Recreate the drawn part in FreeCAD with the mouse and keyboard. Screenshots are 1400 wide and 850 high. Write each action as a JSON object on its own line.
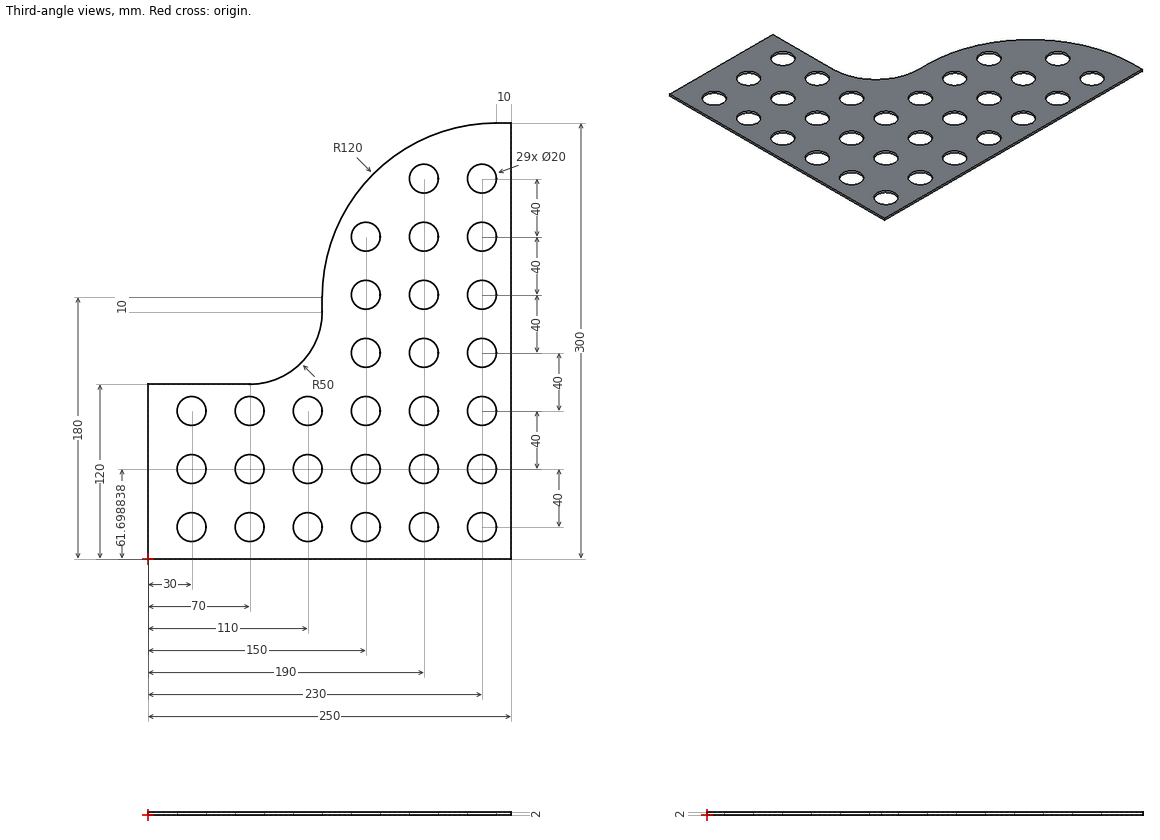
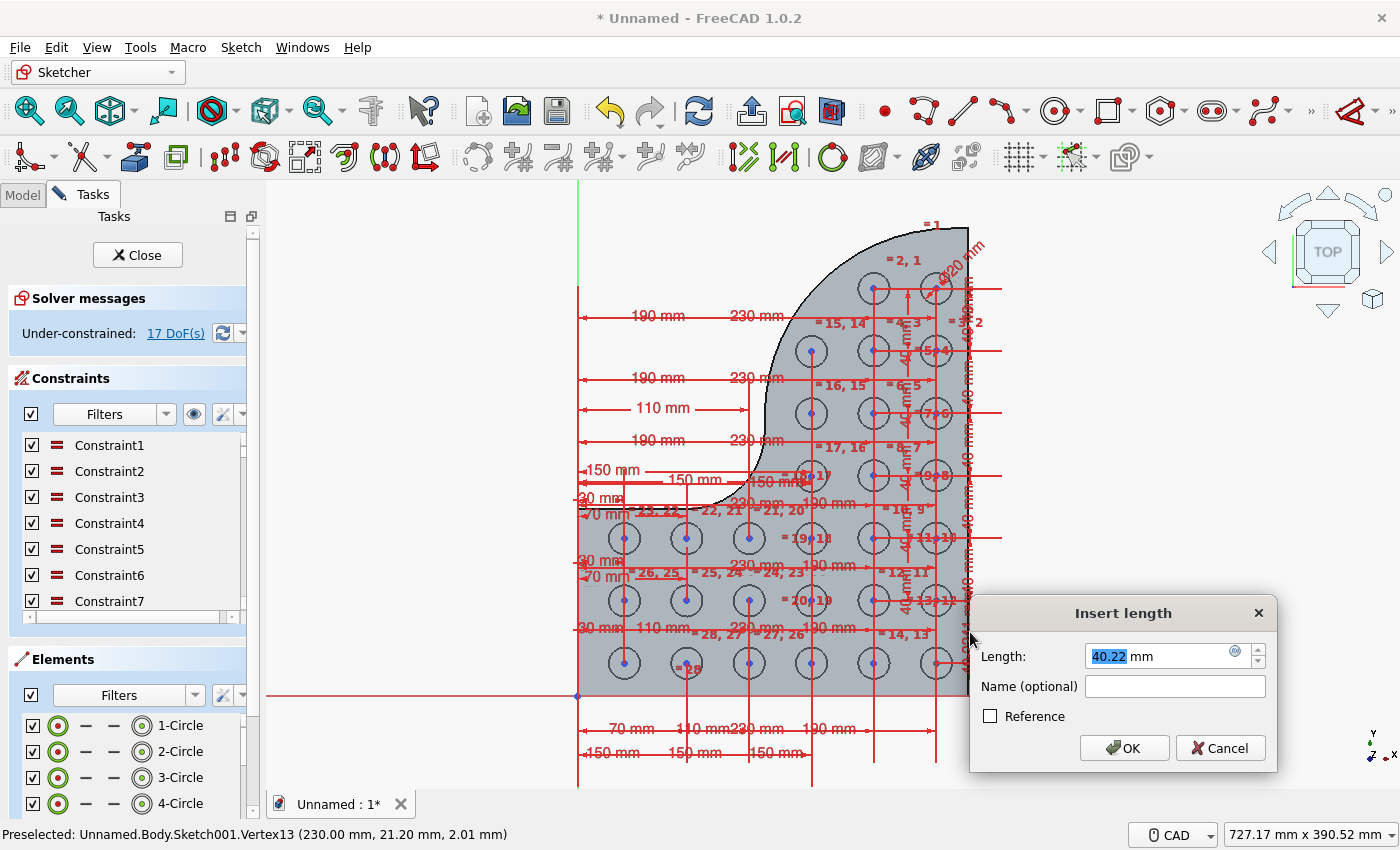
{"action": "type", "text": "40"}
{"action": "key", "text": "Return"}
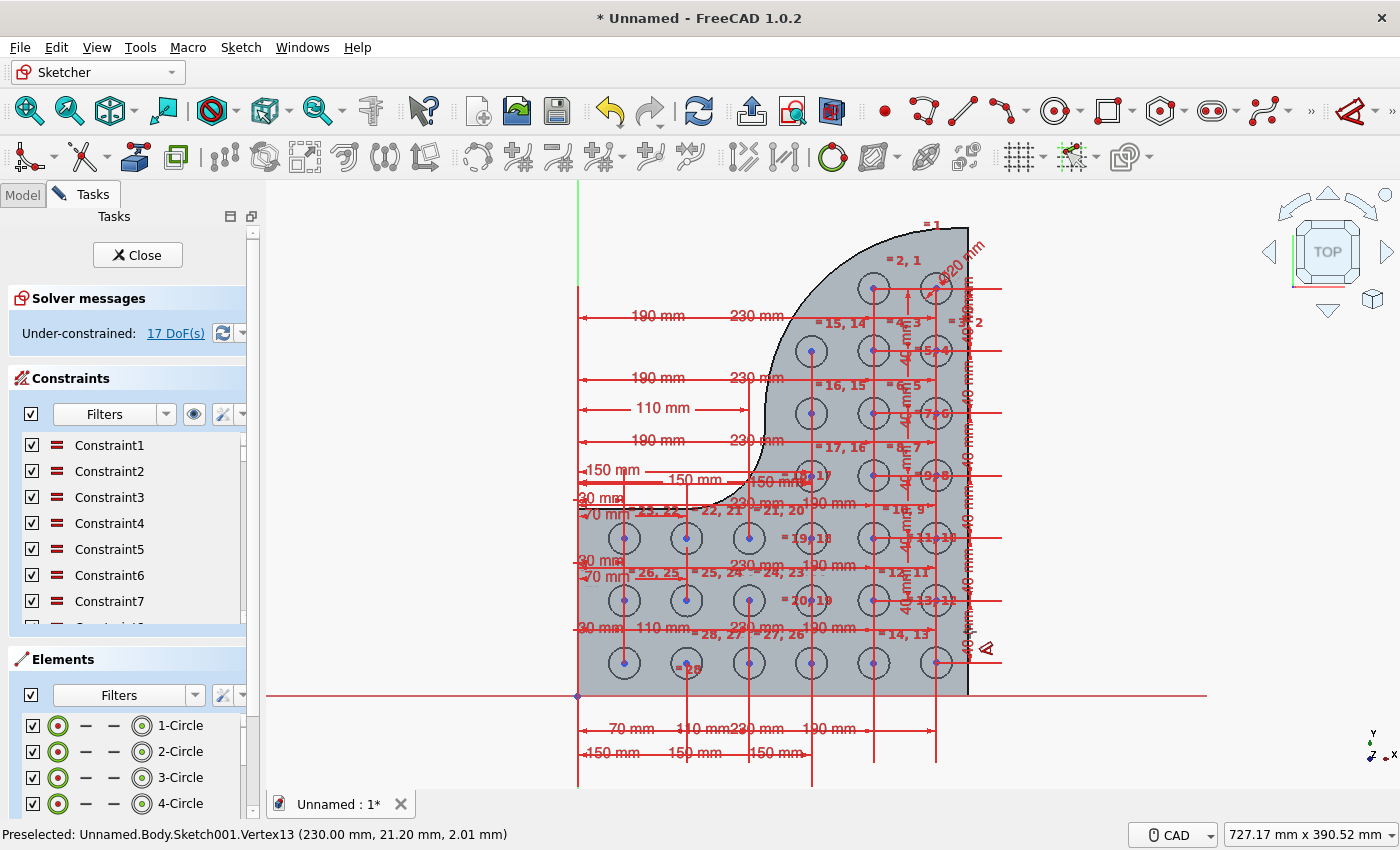
{"action": "left_click", "coordinate": [874, 601]}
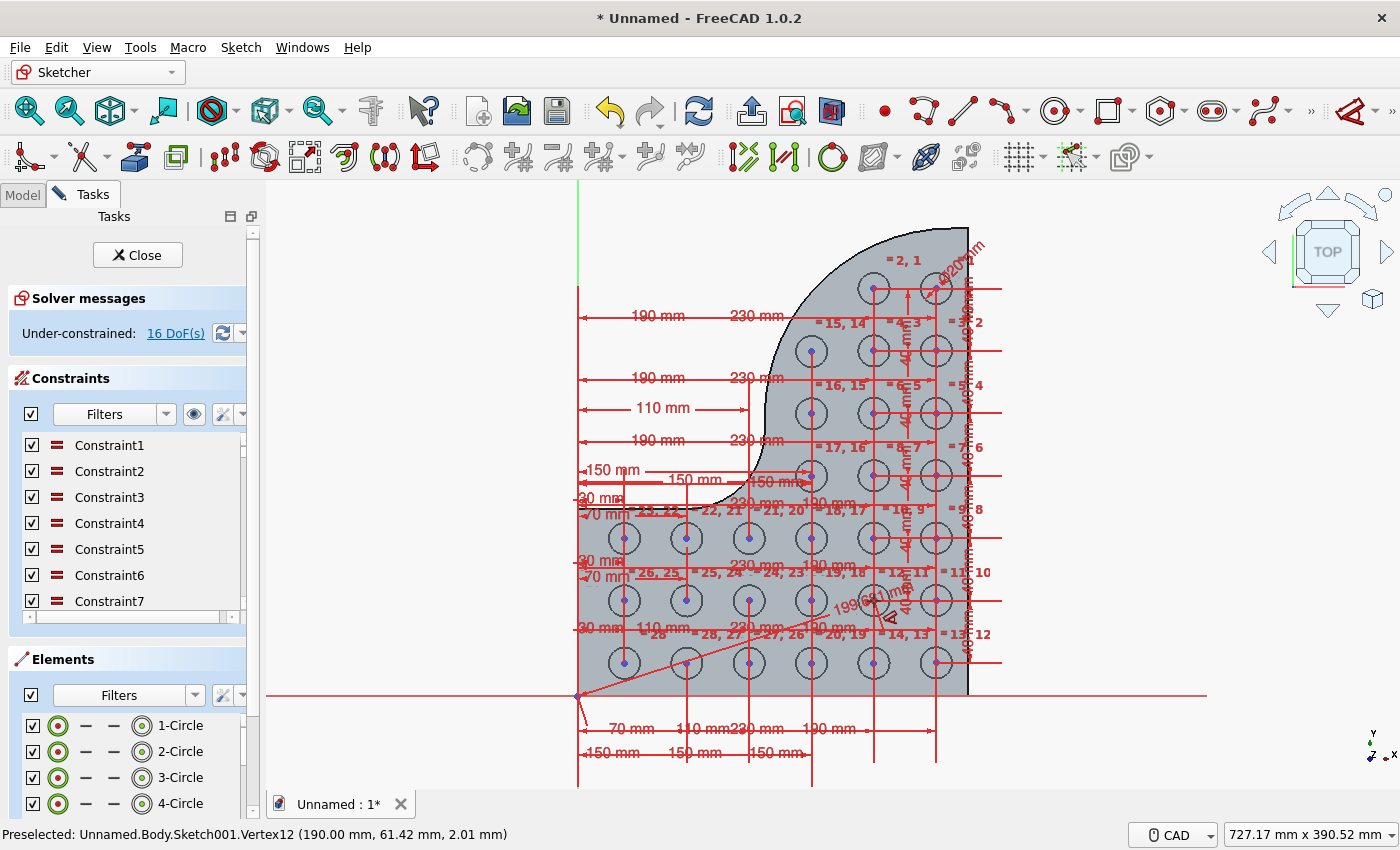
{"action": "left_click", "coordinate": [874, 663]}
{"action": "left_click", "coordinate": [908, 654]}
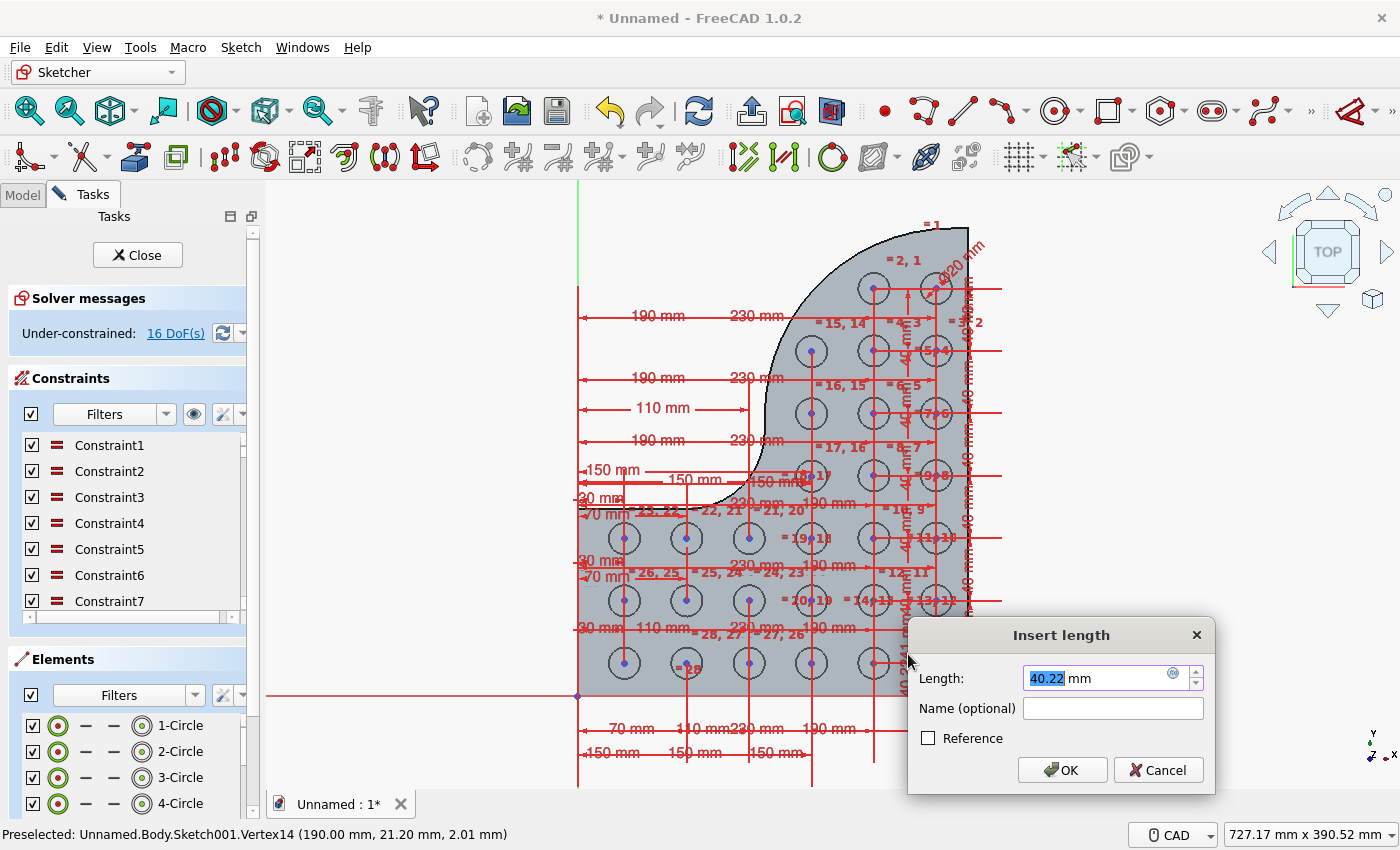
{"action": "type", "text": "40"}
{"action": "key", "text": "Return"}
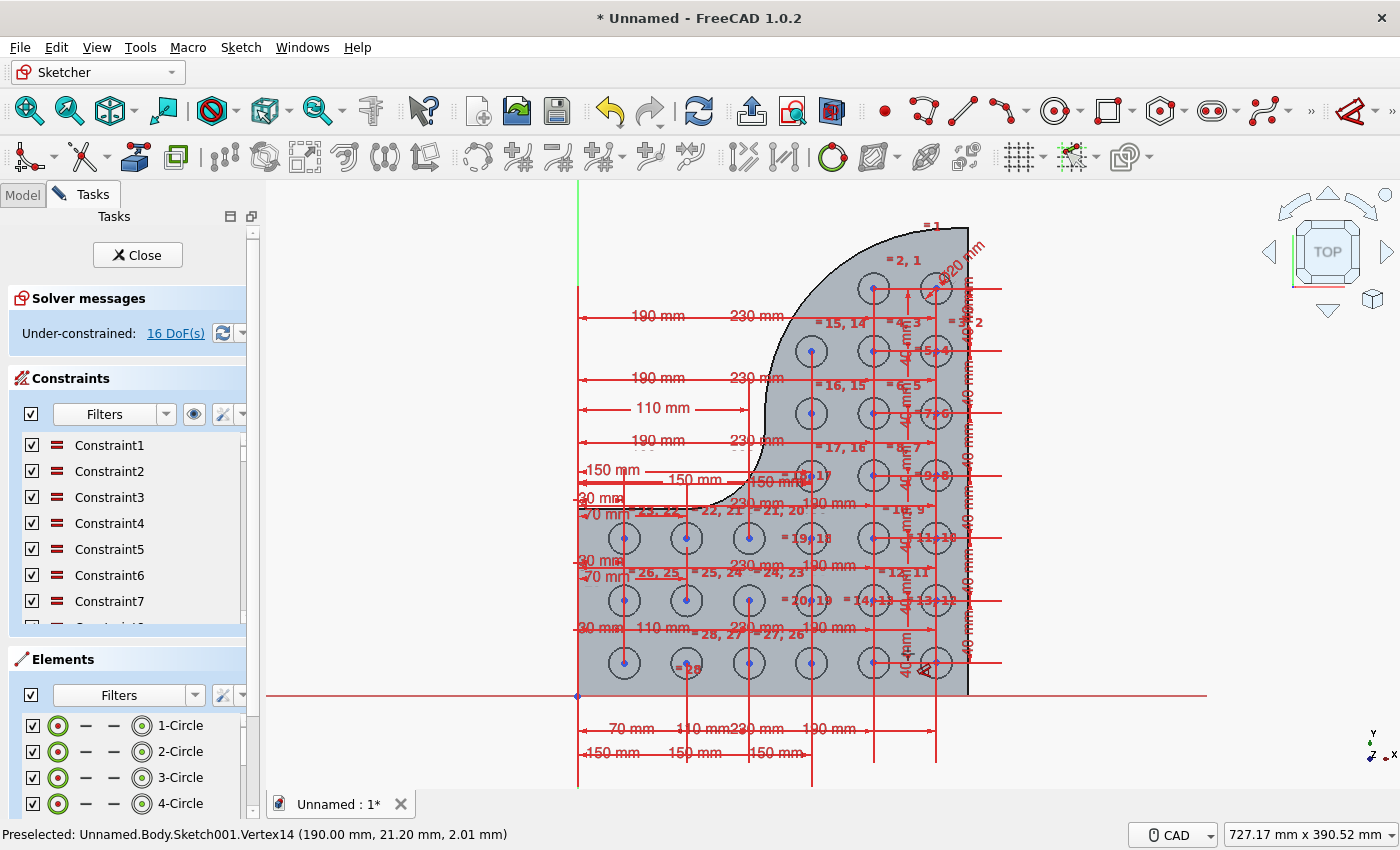
{"action": "left_click", "coordinate": [874, 289]}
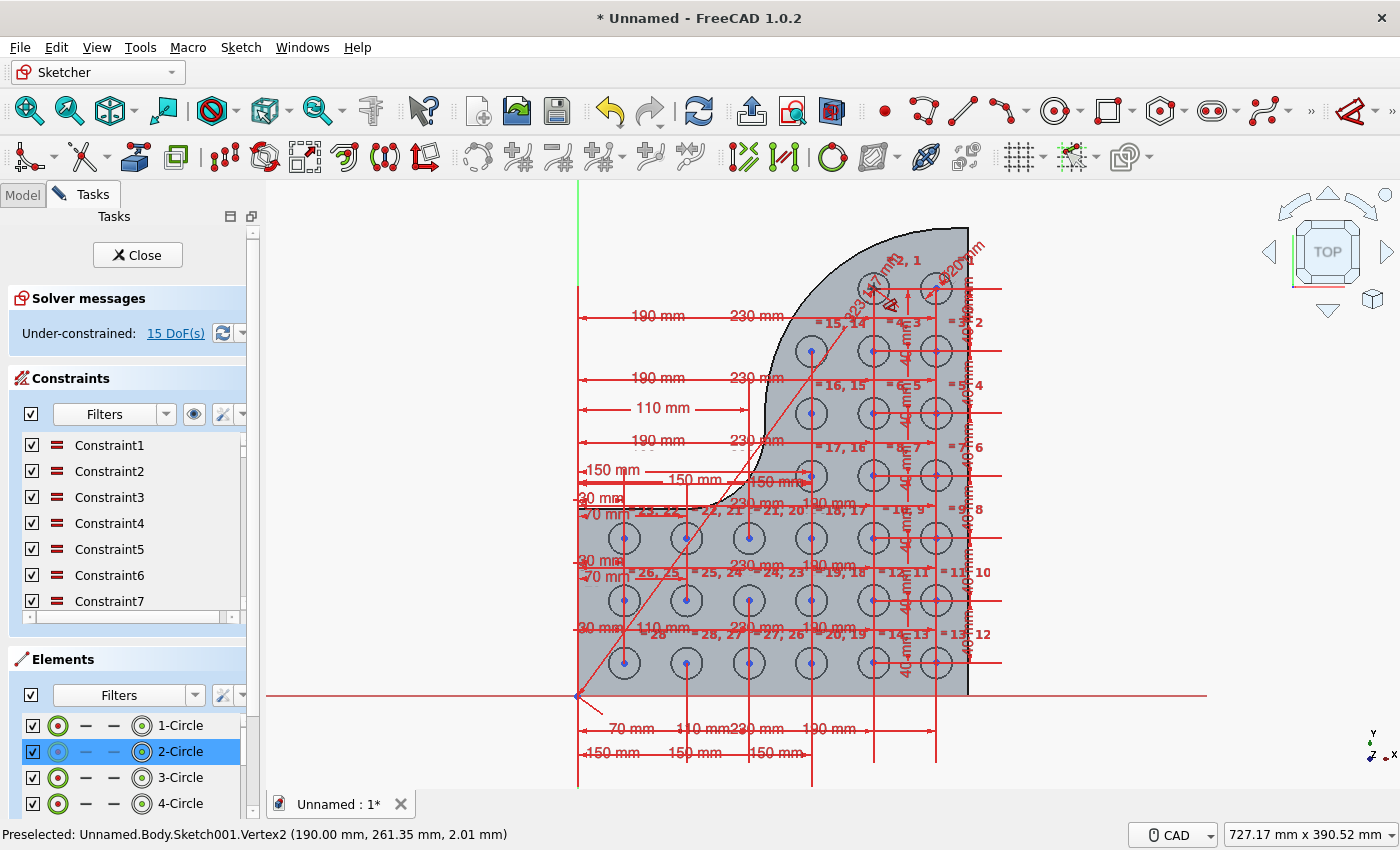
{"action": "left_click", "coordinate": [812, 352]}
{"action": "left_click", "coordinate": [778, 342]}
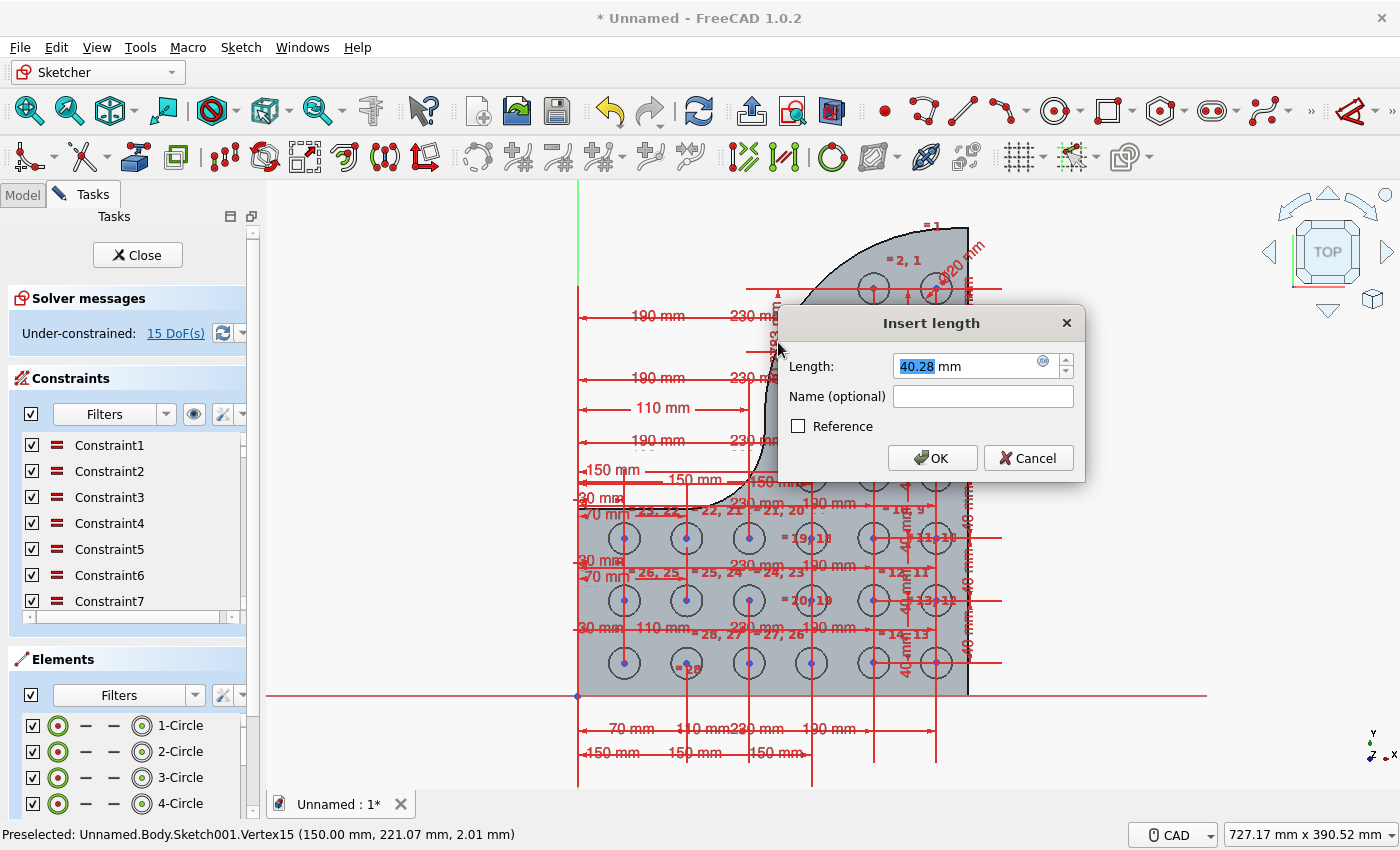
{"action": "type", "text": "40"}
{"action": "key", "text": "Return"}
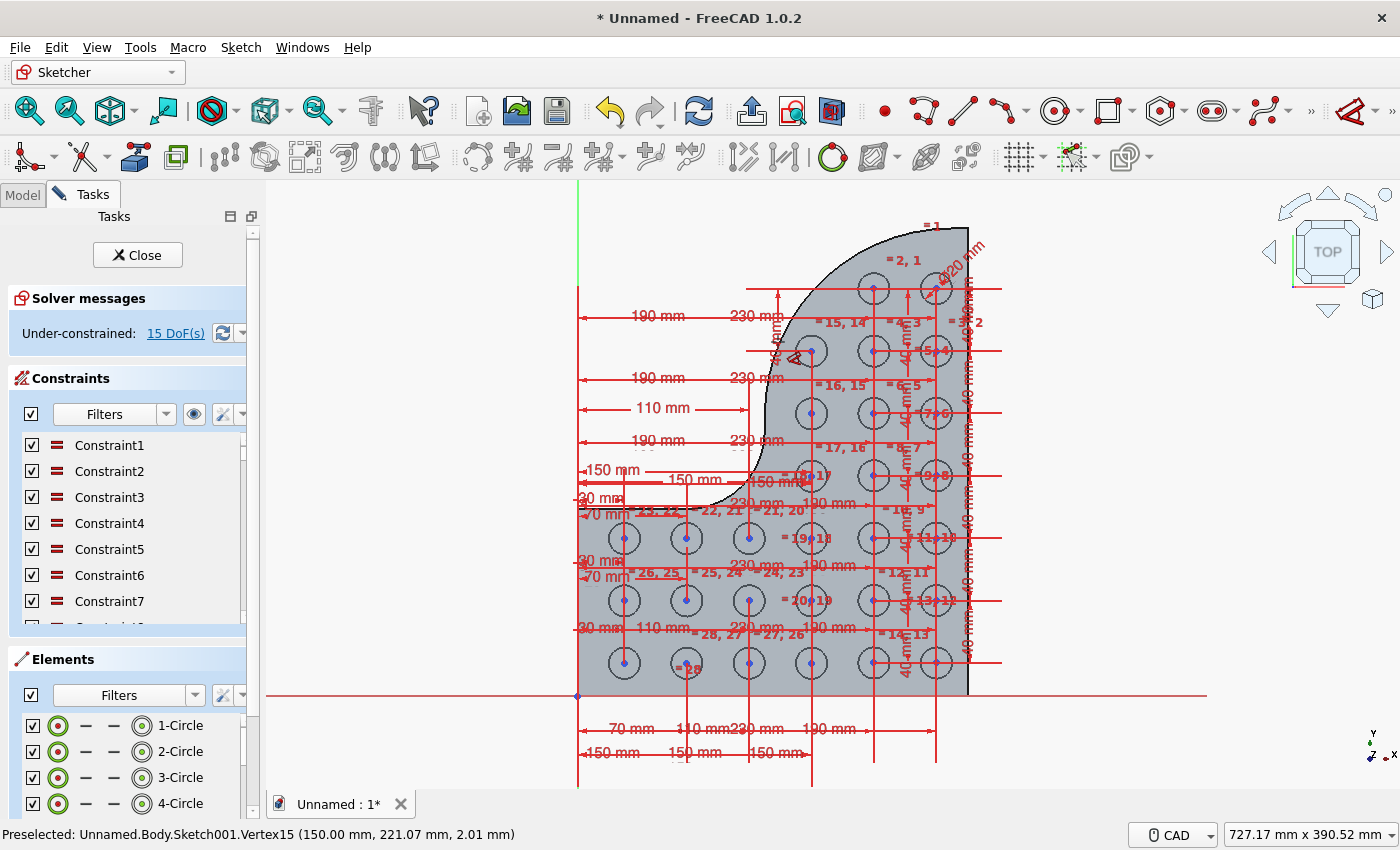
{"action": "left_click", "coordinate": [812, 351]}